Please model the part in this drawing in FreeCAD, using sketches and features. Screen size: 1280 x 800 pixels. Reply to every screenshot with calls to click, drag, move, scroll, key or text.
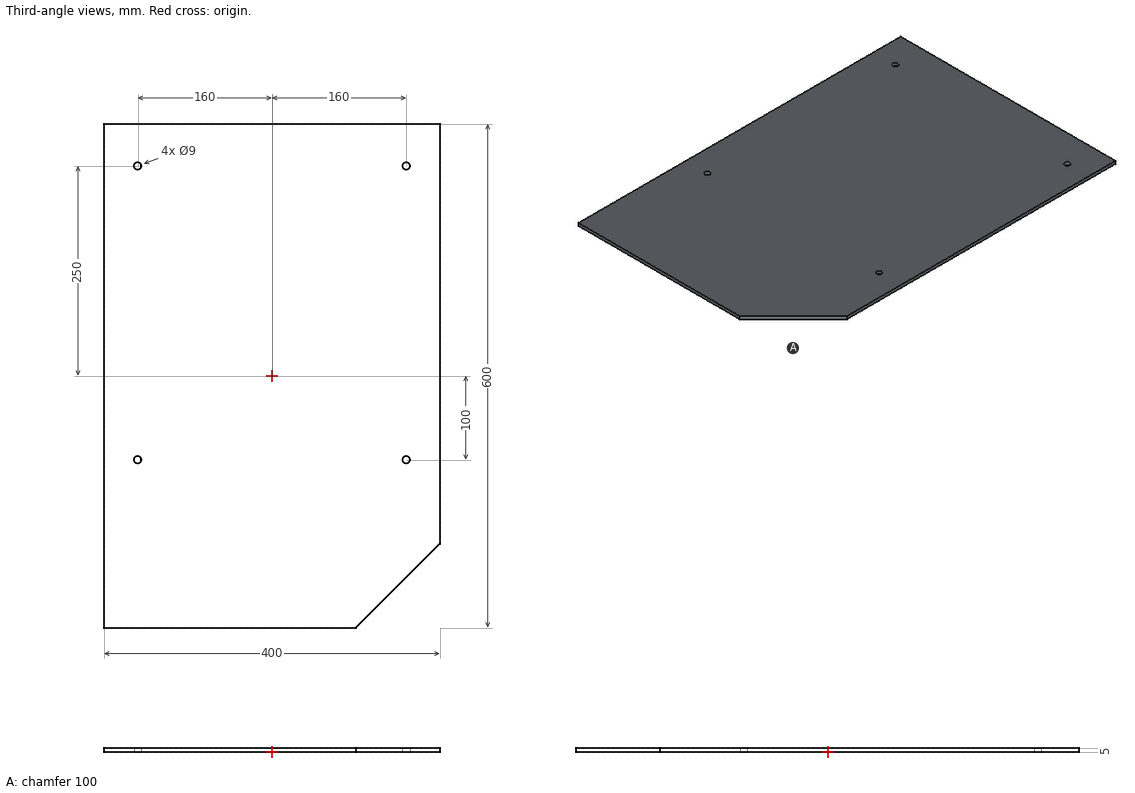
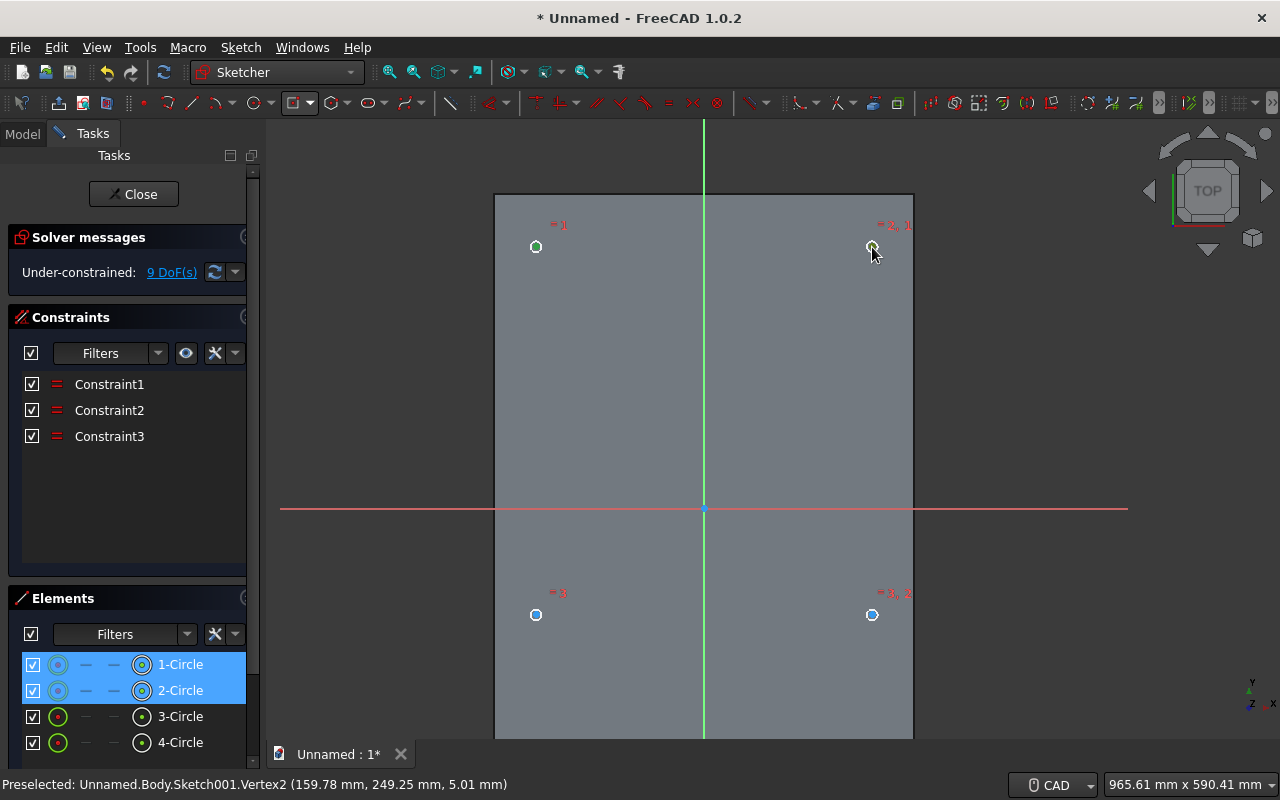
click(578, 104)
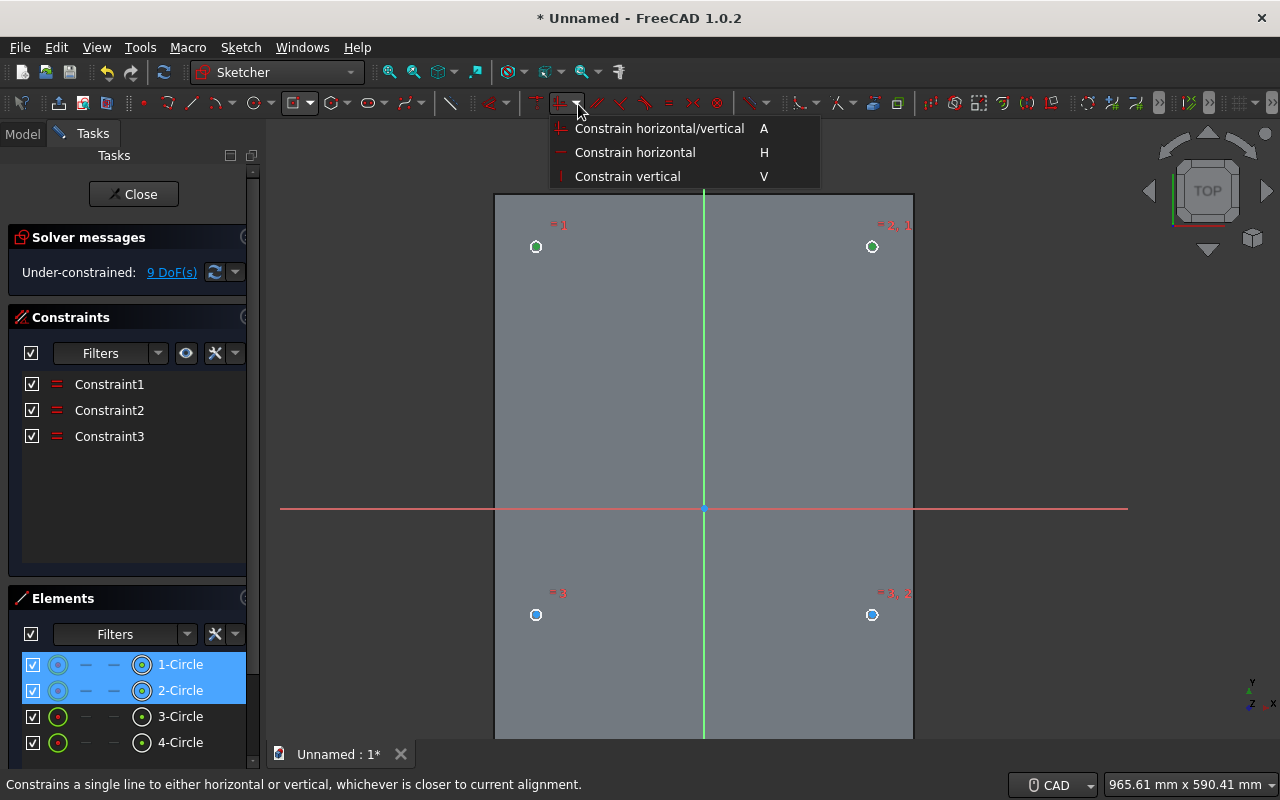
click(685, 152)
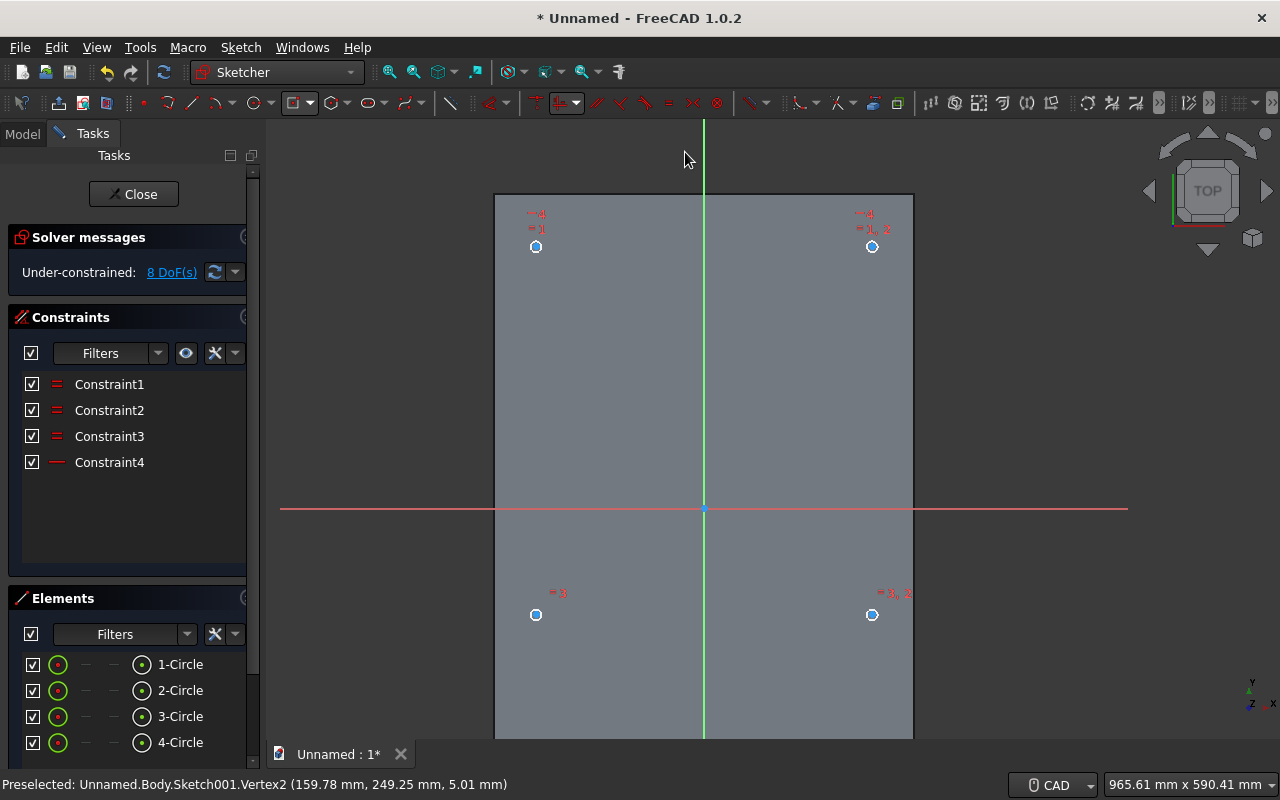
click(872, 247)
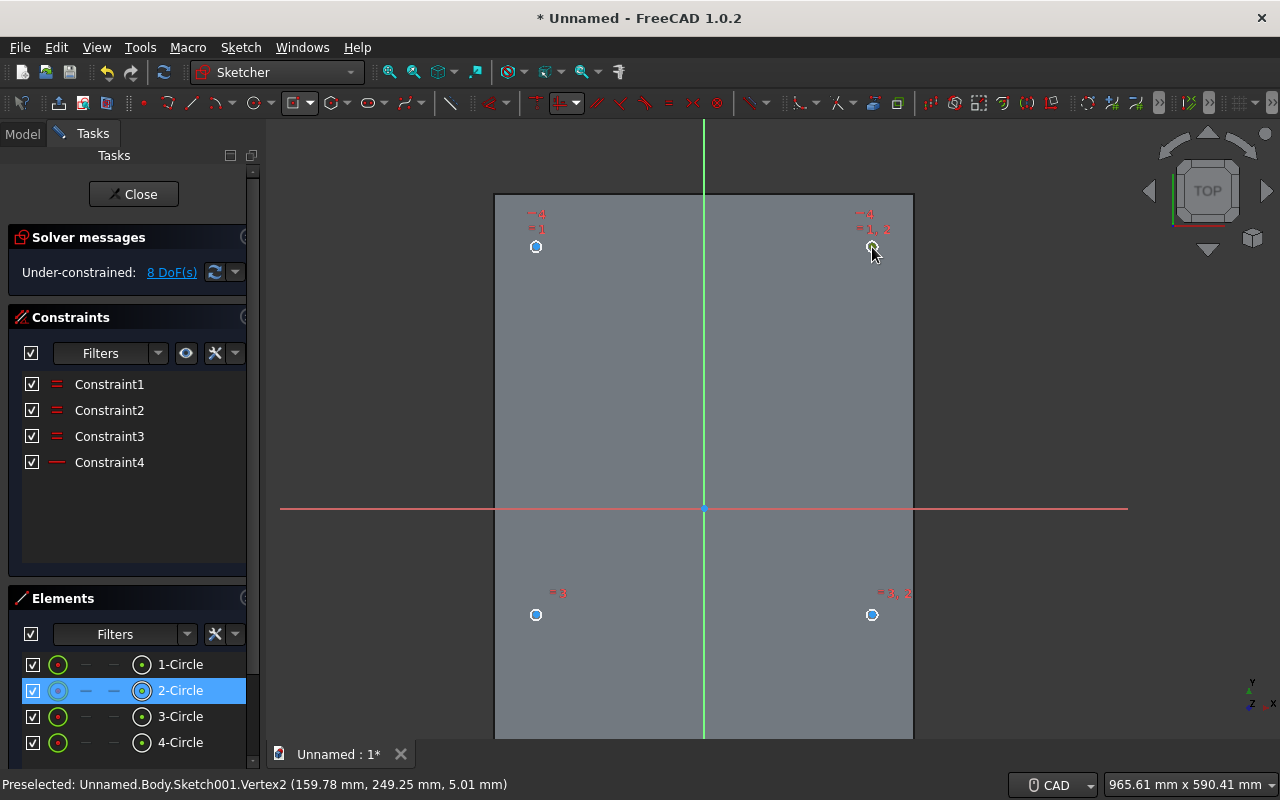
click(872, 615)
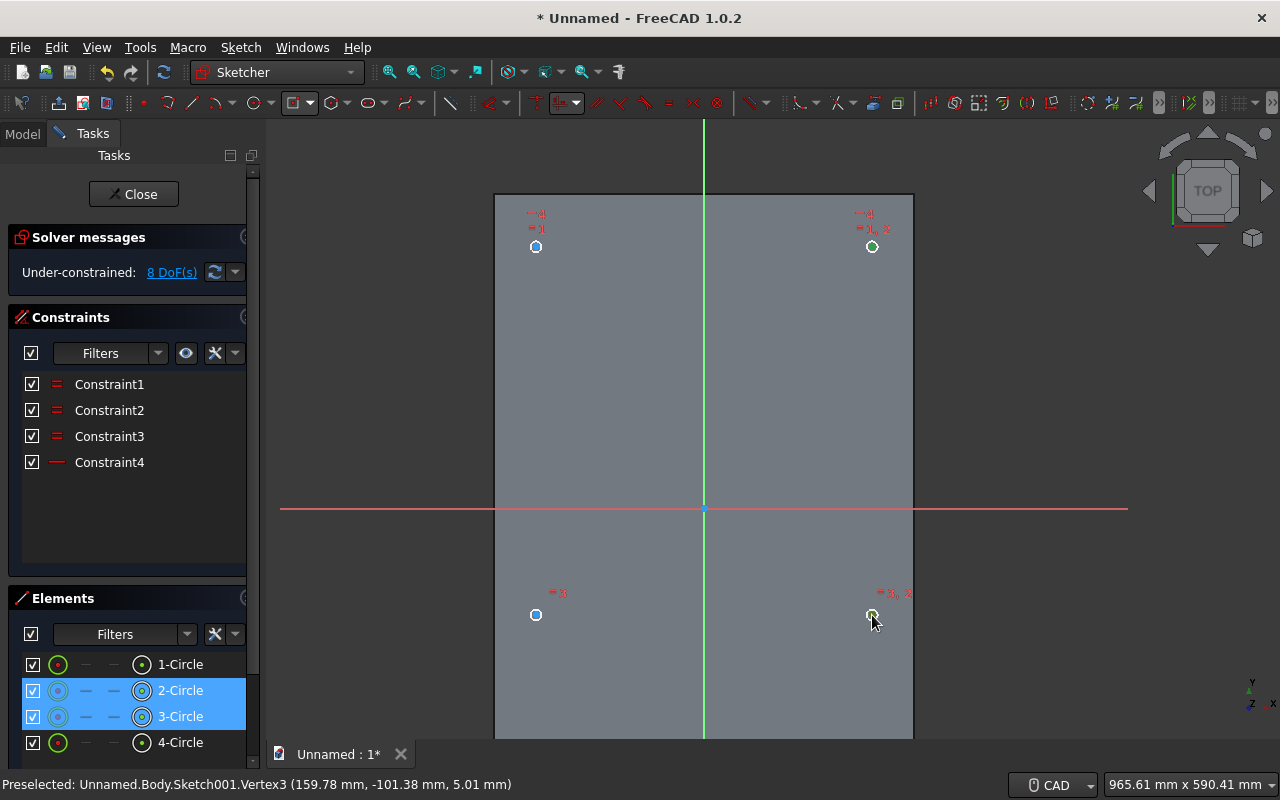
click(578, 104)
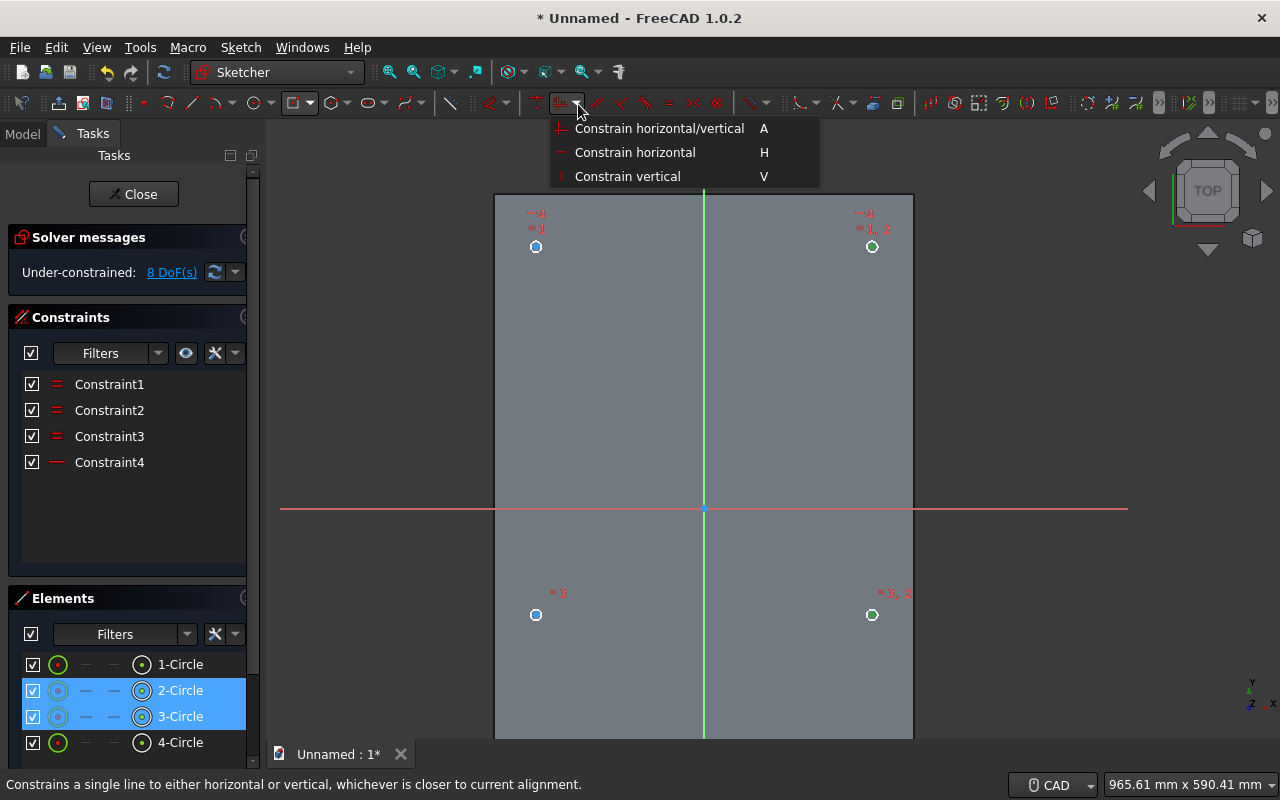
click(685, 176)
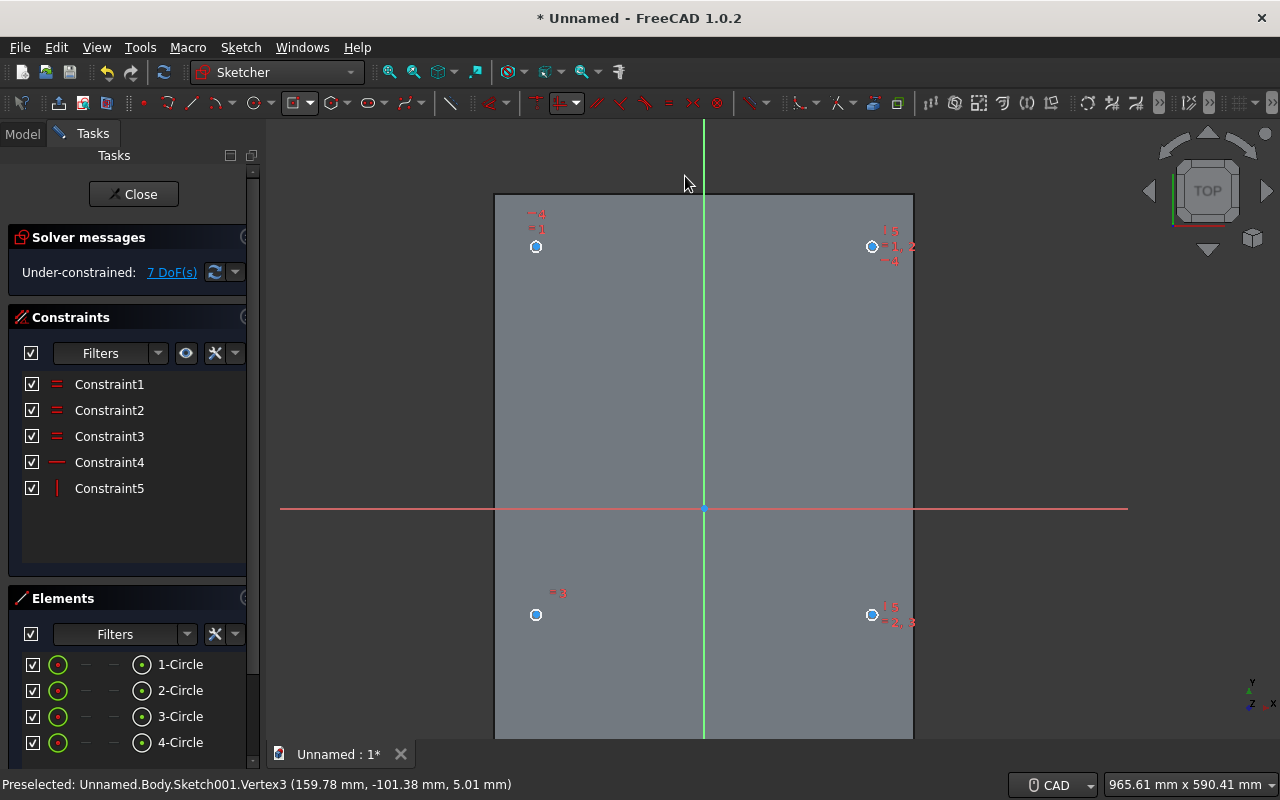
click(536, 247)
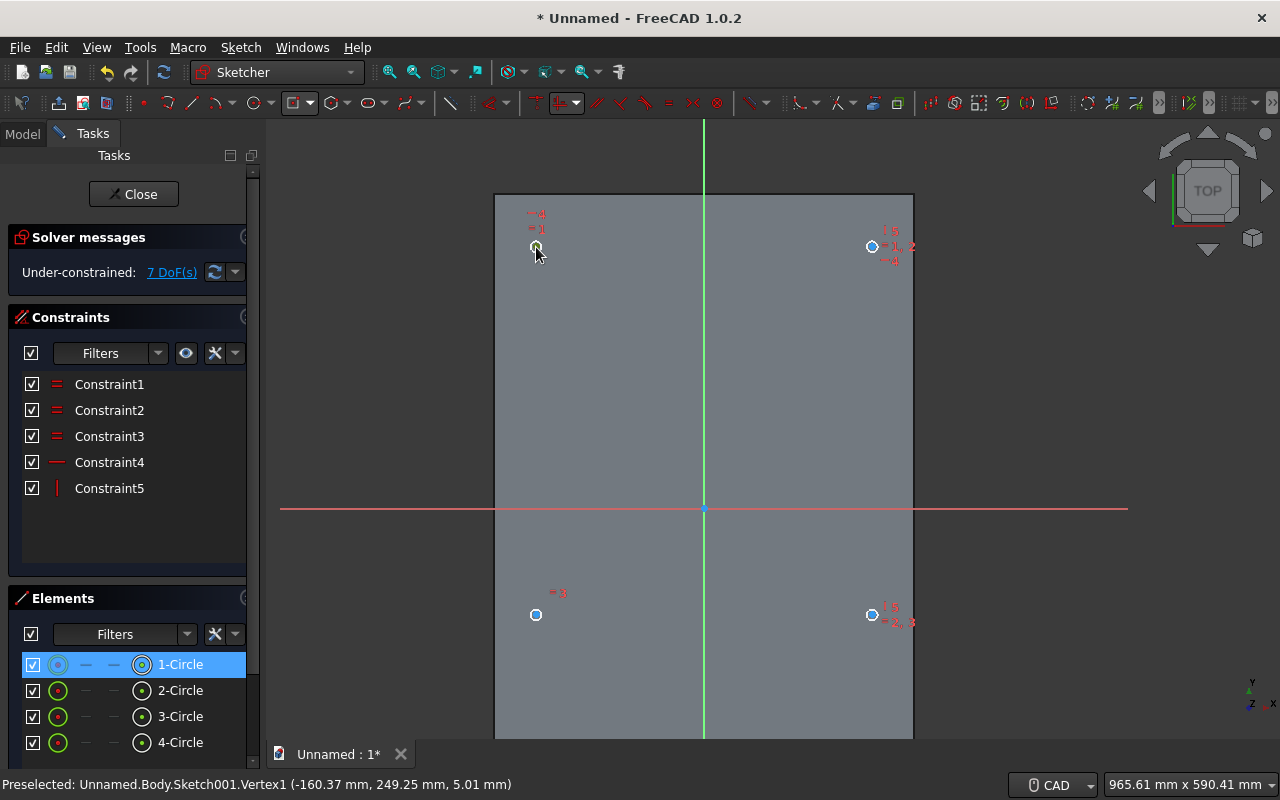
click(536, 615)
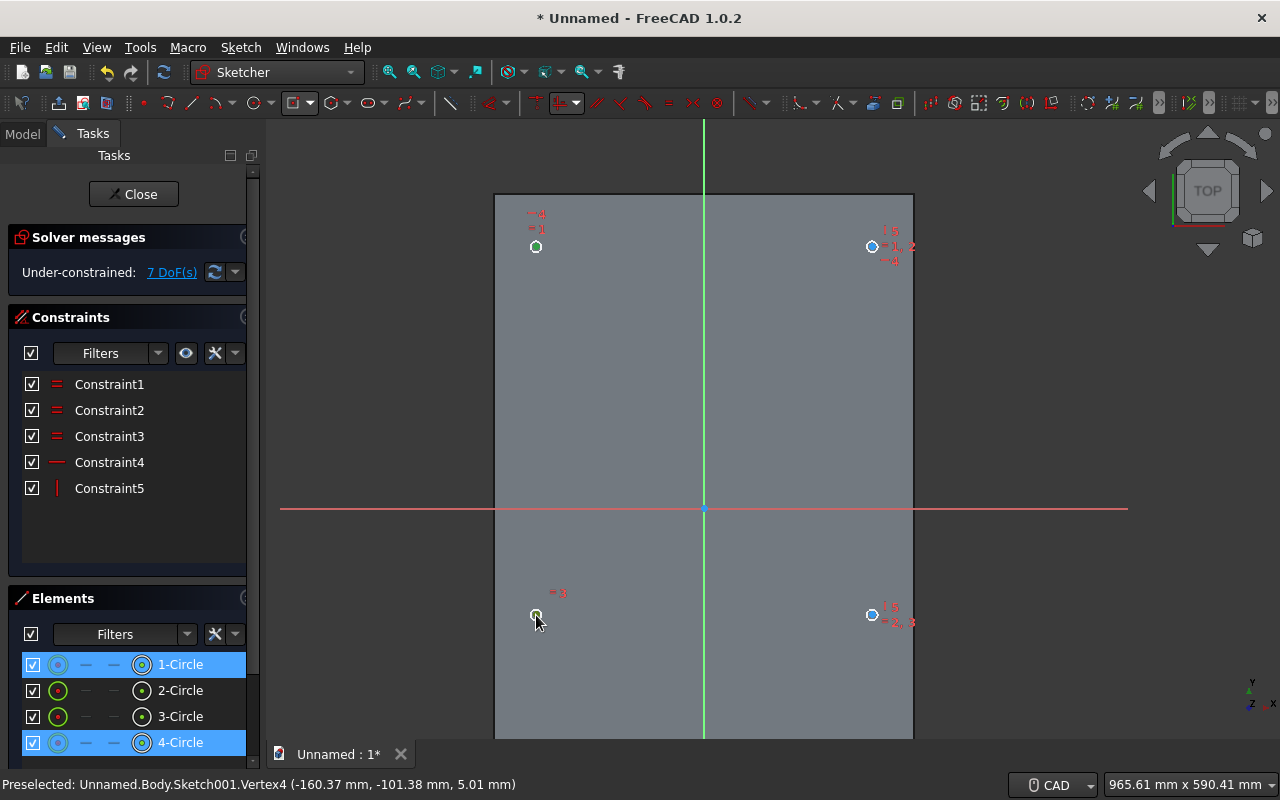
key(v)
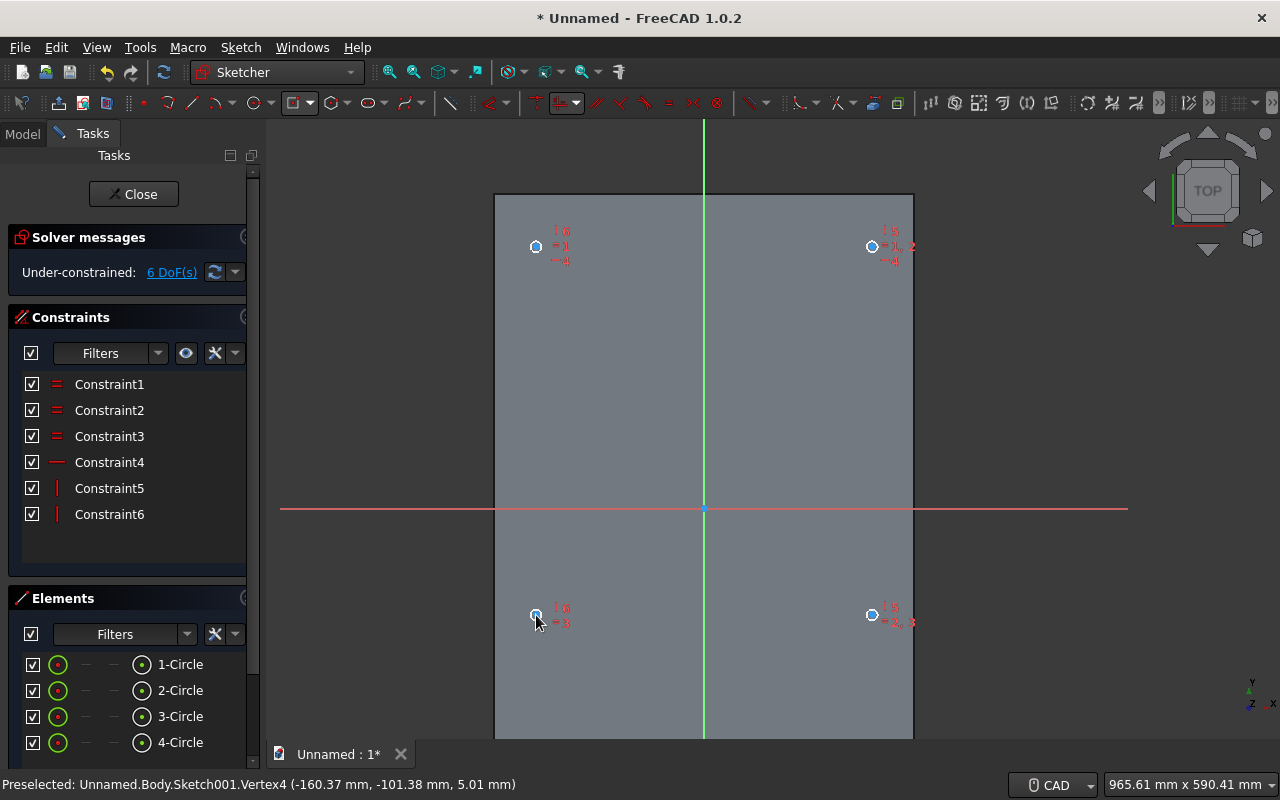
click(872, 615)